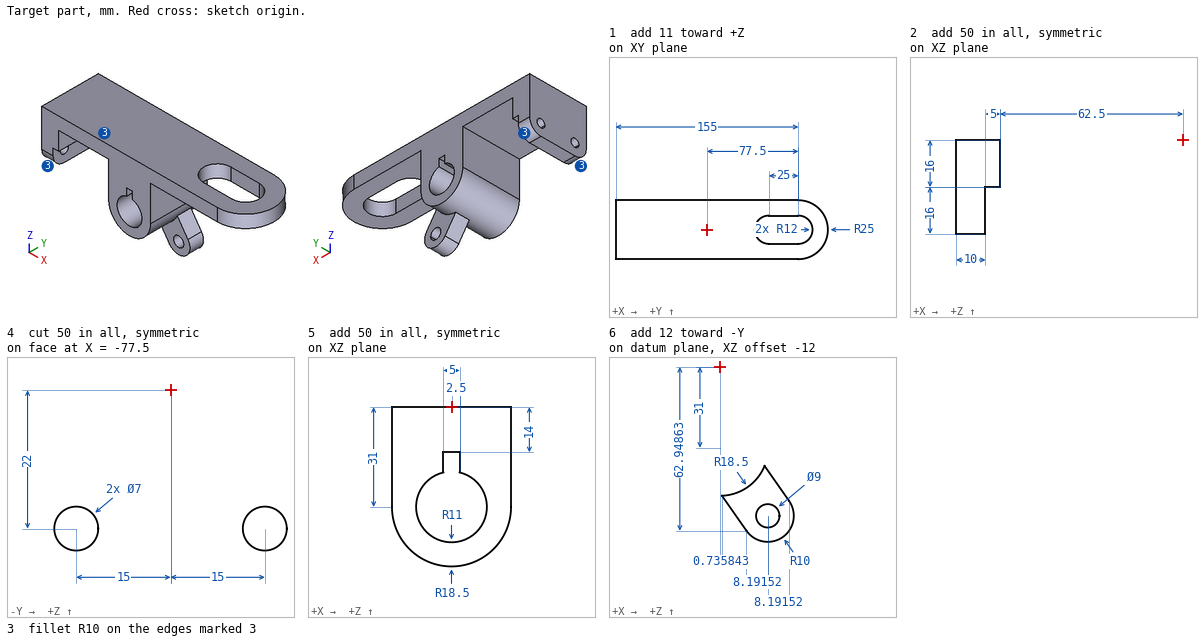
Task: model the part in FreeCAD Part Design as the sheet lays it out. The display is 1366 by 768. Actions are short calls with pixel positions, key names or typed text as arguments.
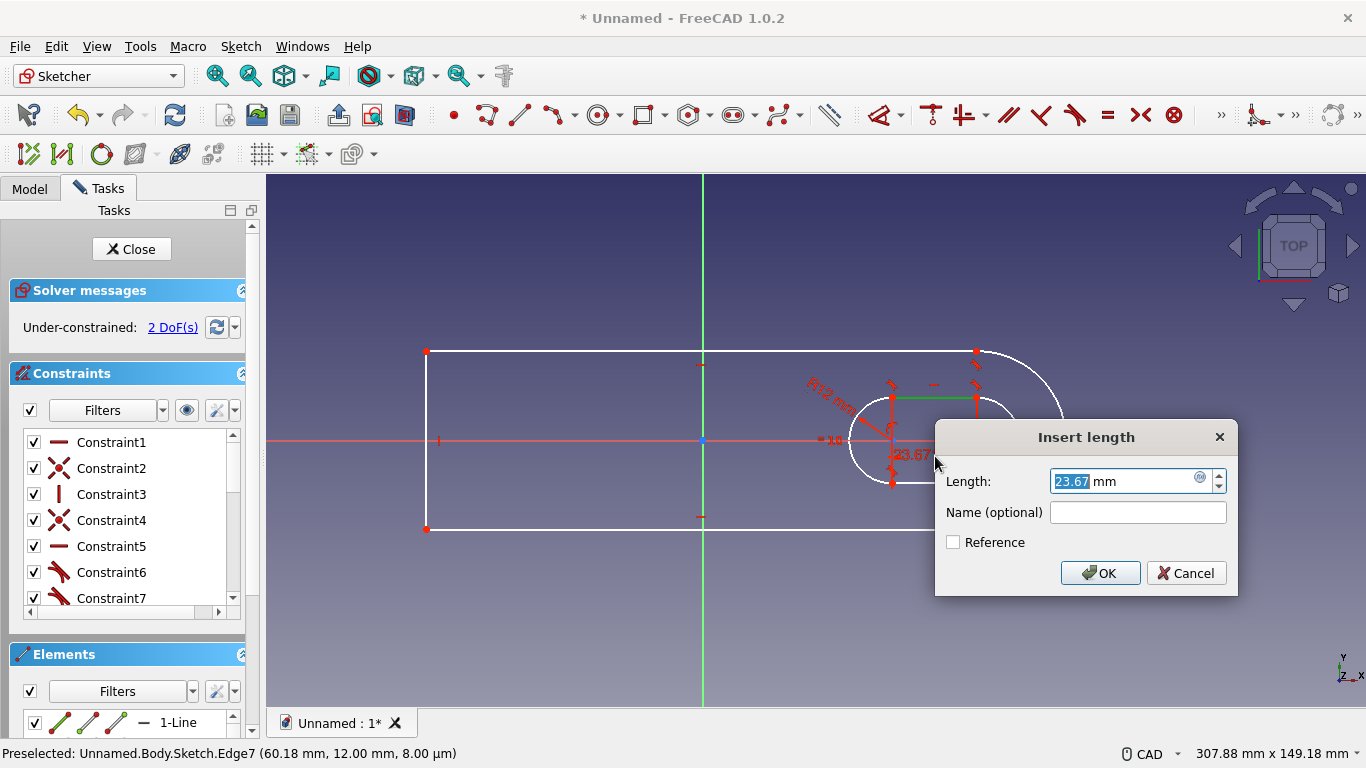
text(25)
key(Return)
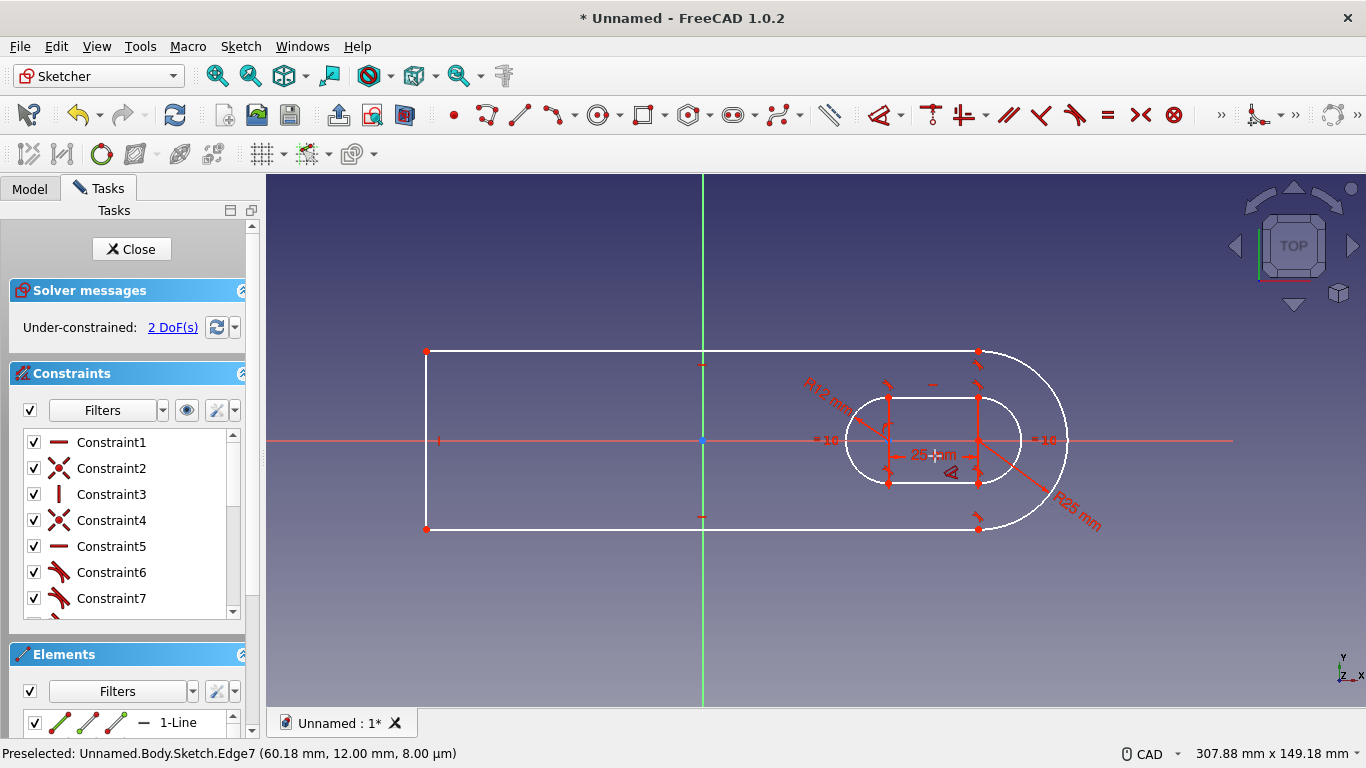
click(813, 351)
click(575, 317)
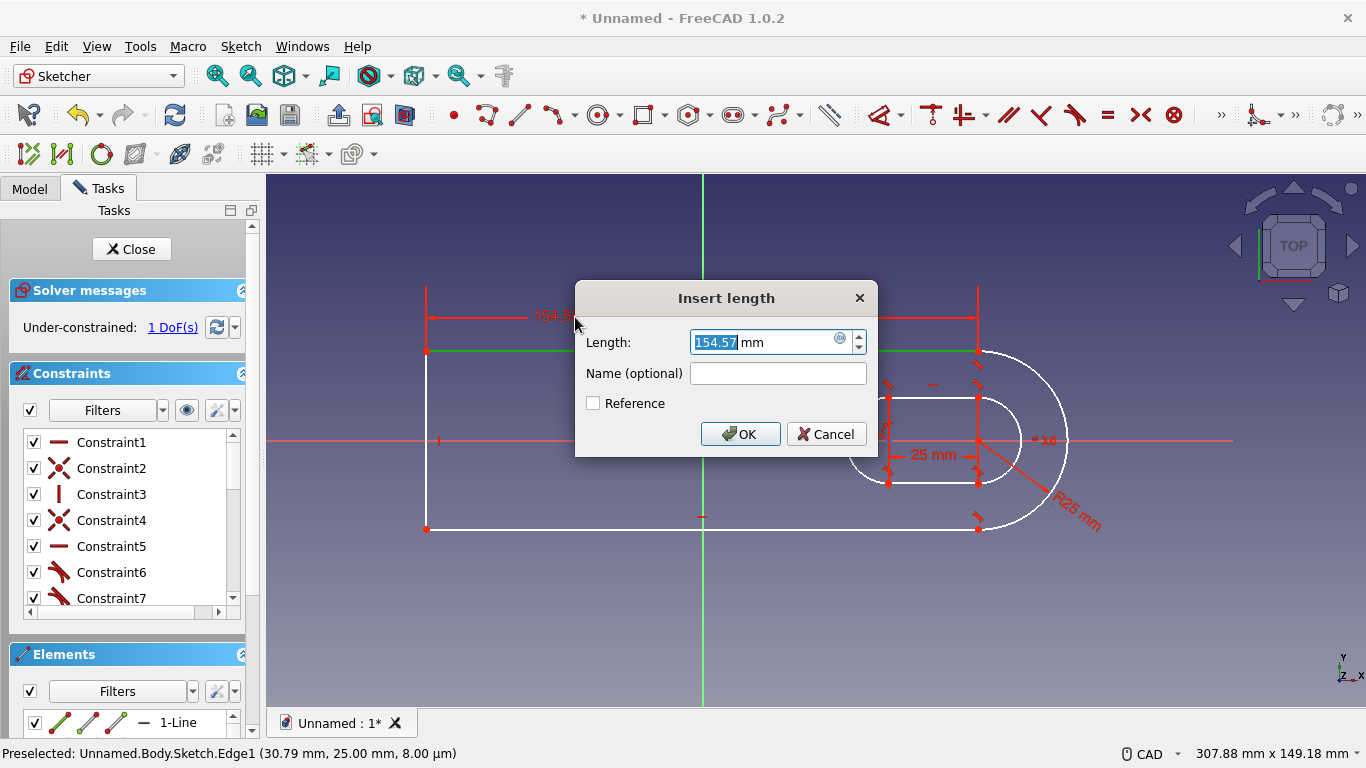
text(155)
key(Return)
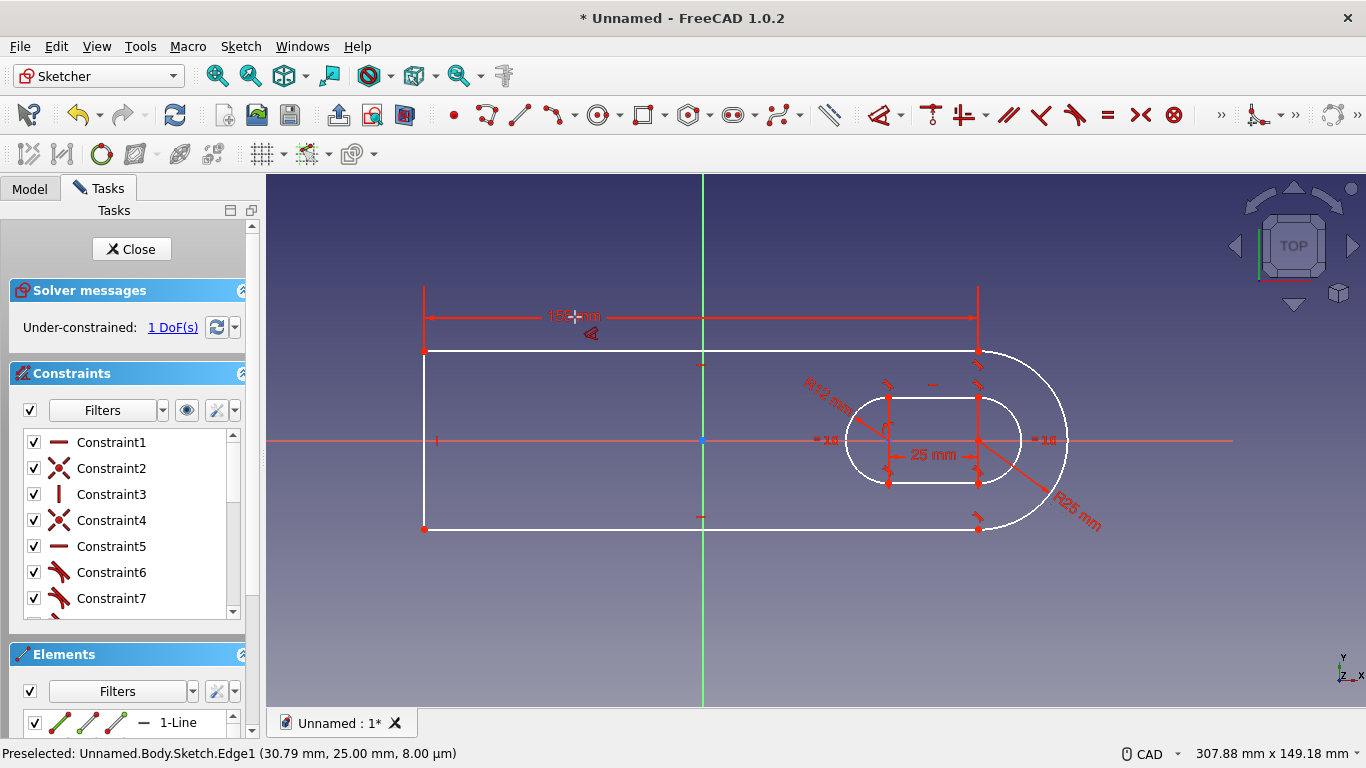
click(978, 351)
click(841, 317)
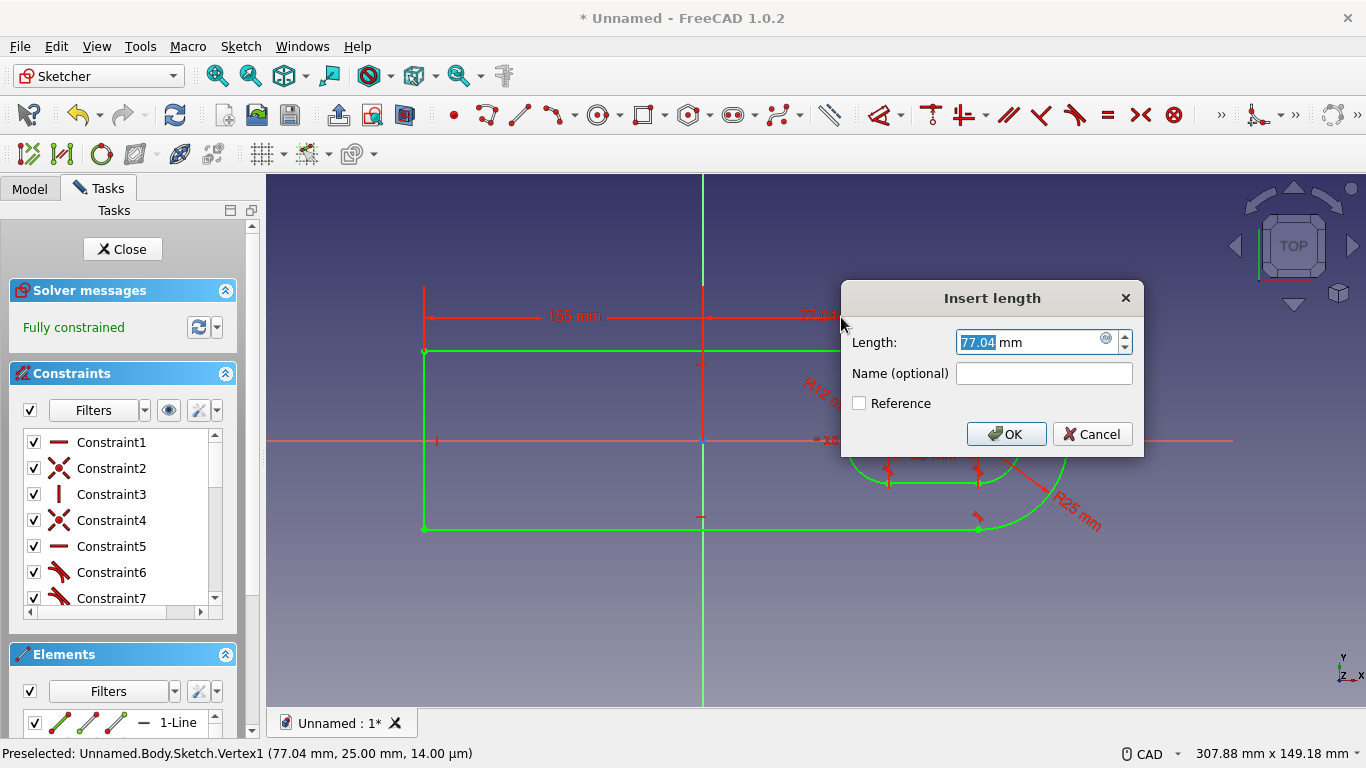
text(77.5)
key(Return)
key(Escape)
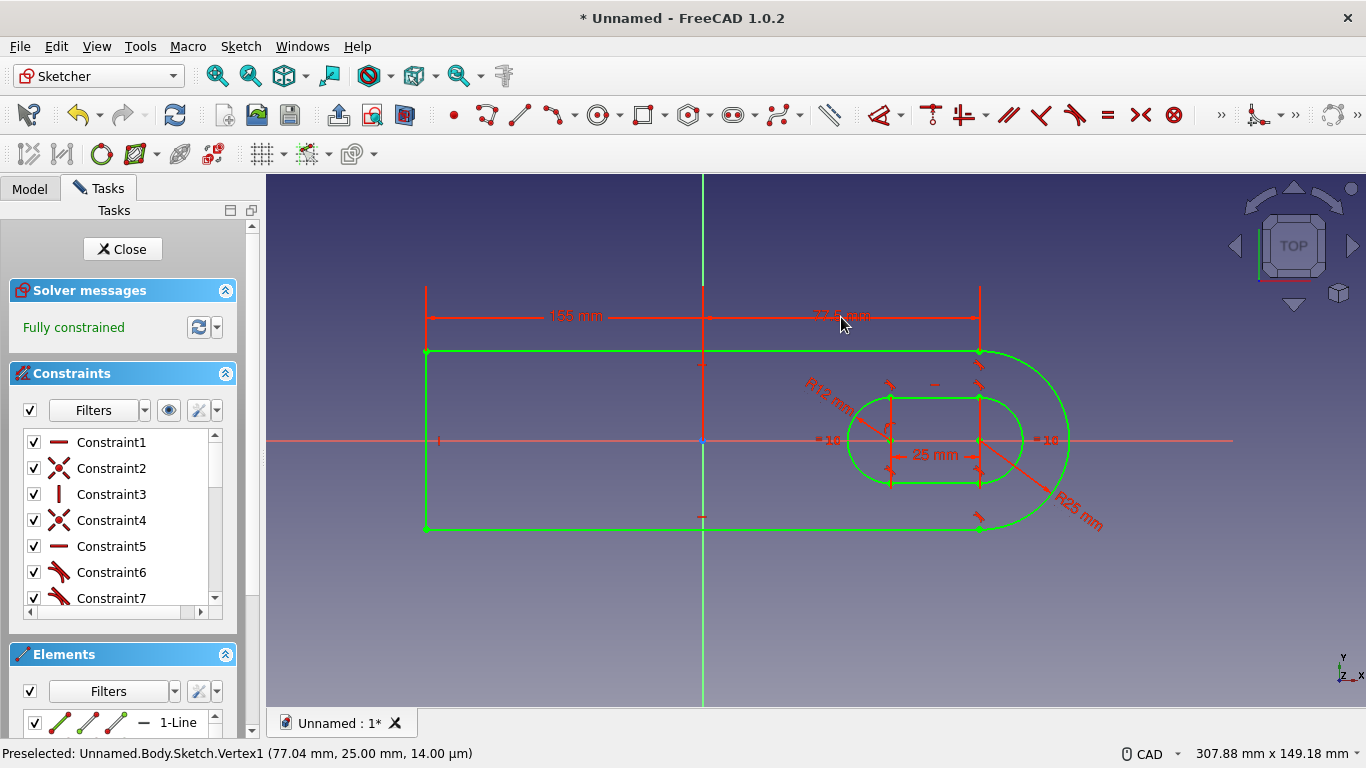
click(123, 249)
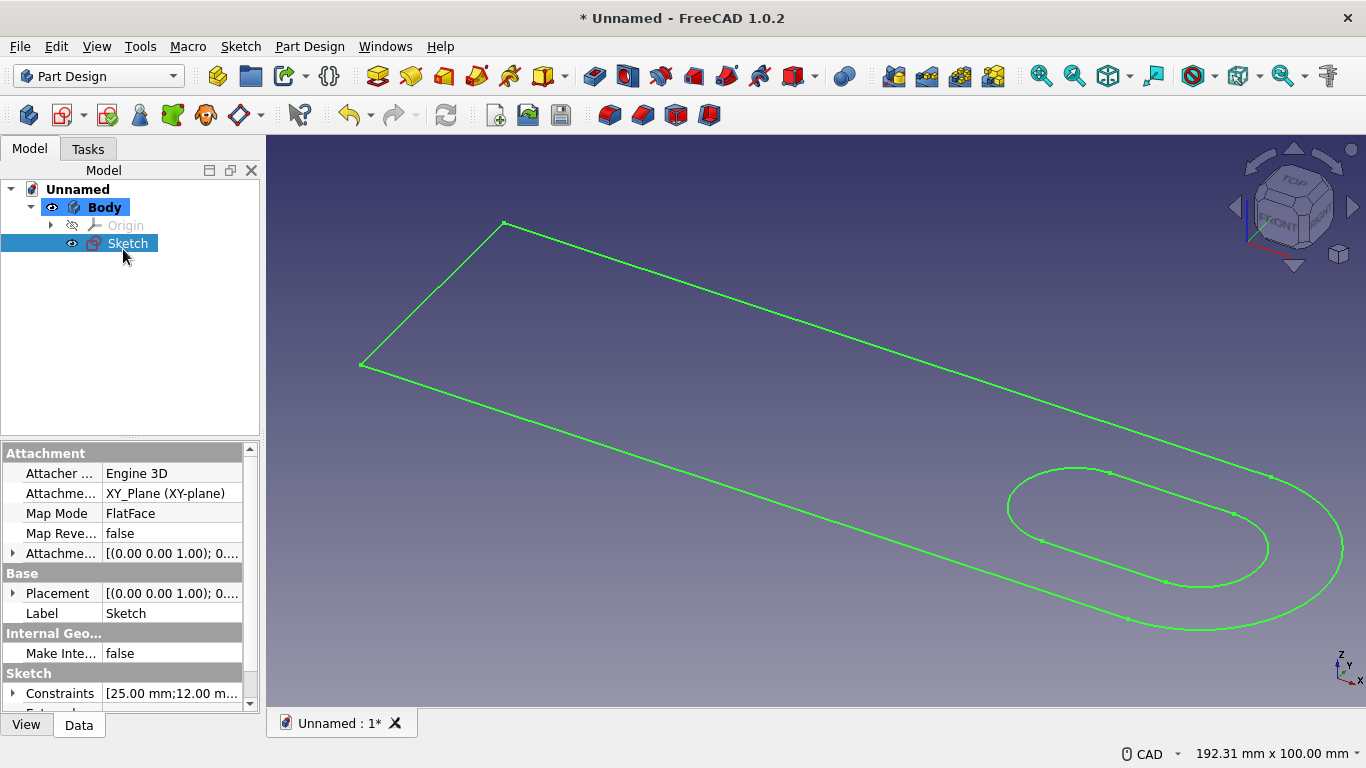
click(378, 76)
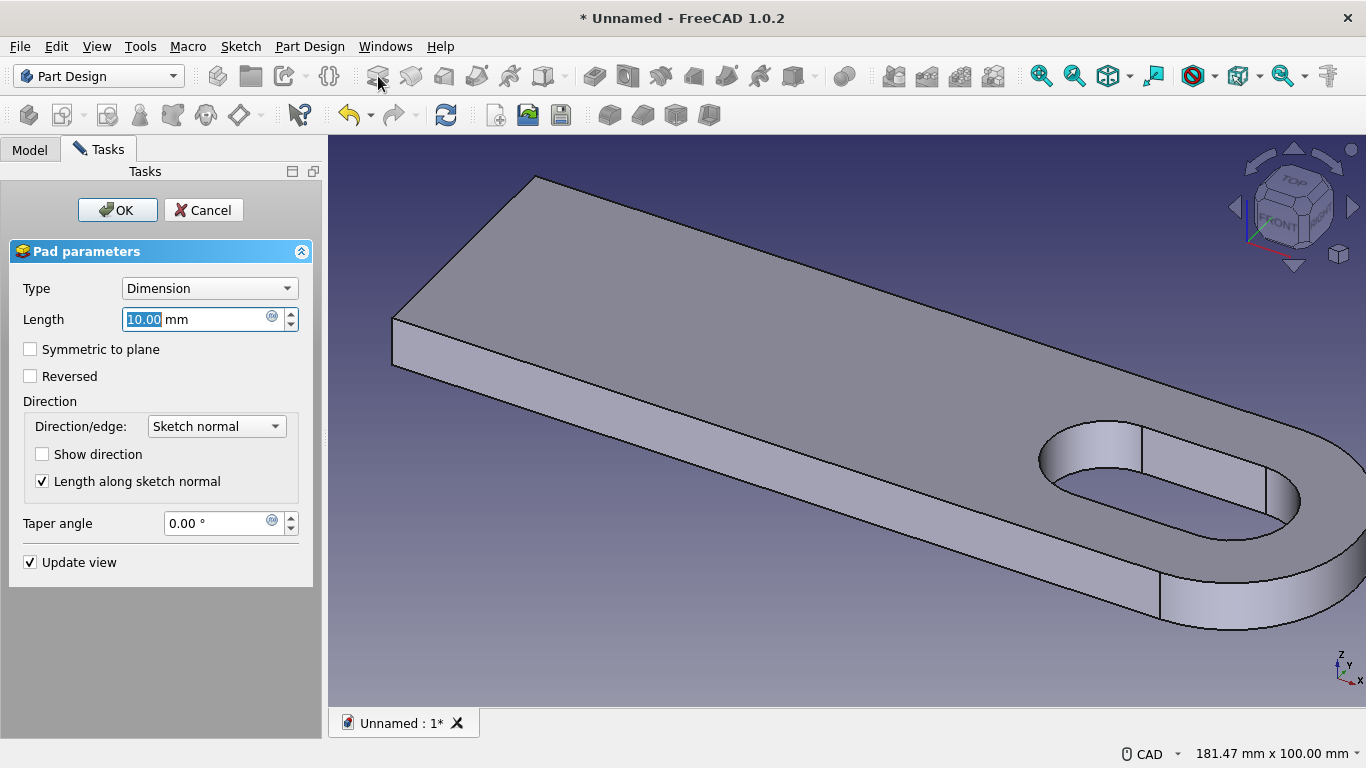
text(11)
key(Tab)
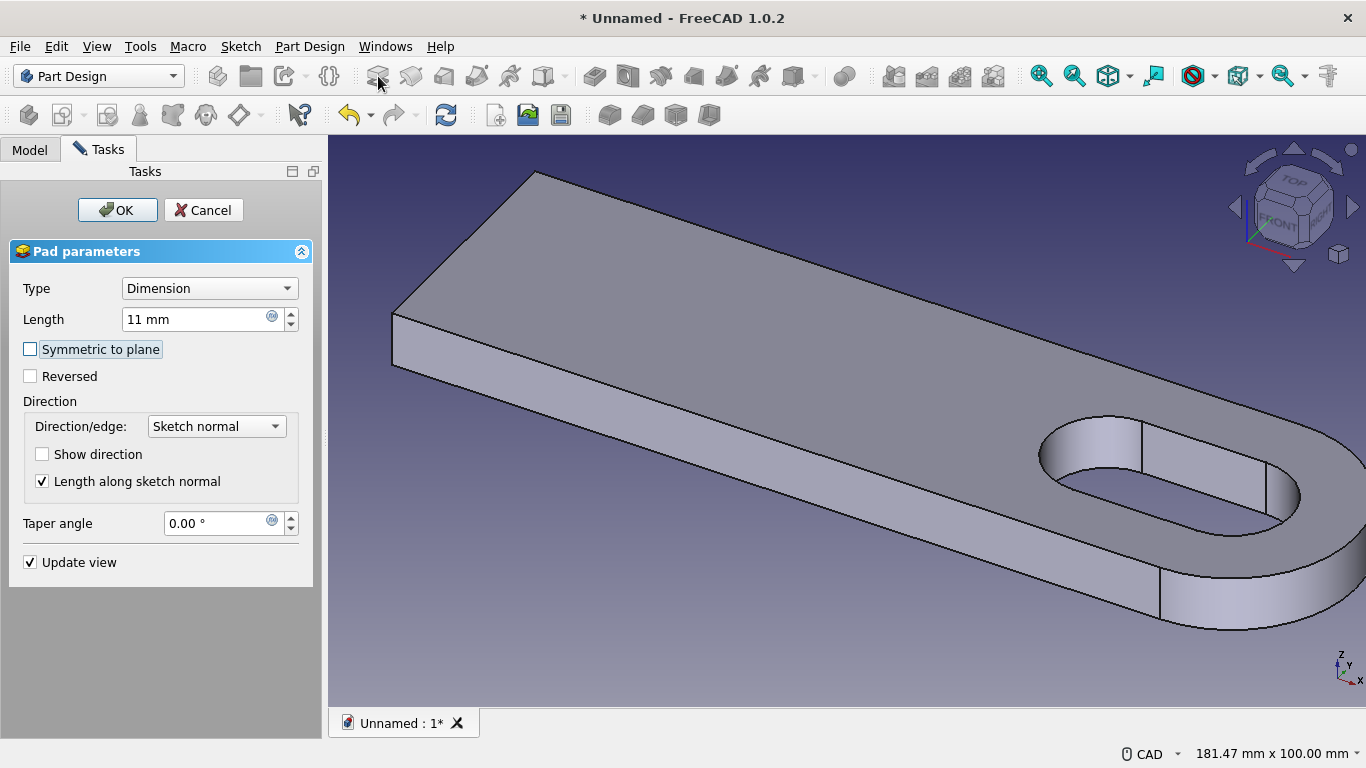
click(118, 210)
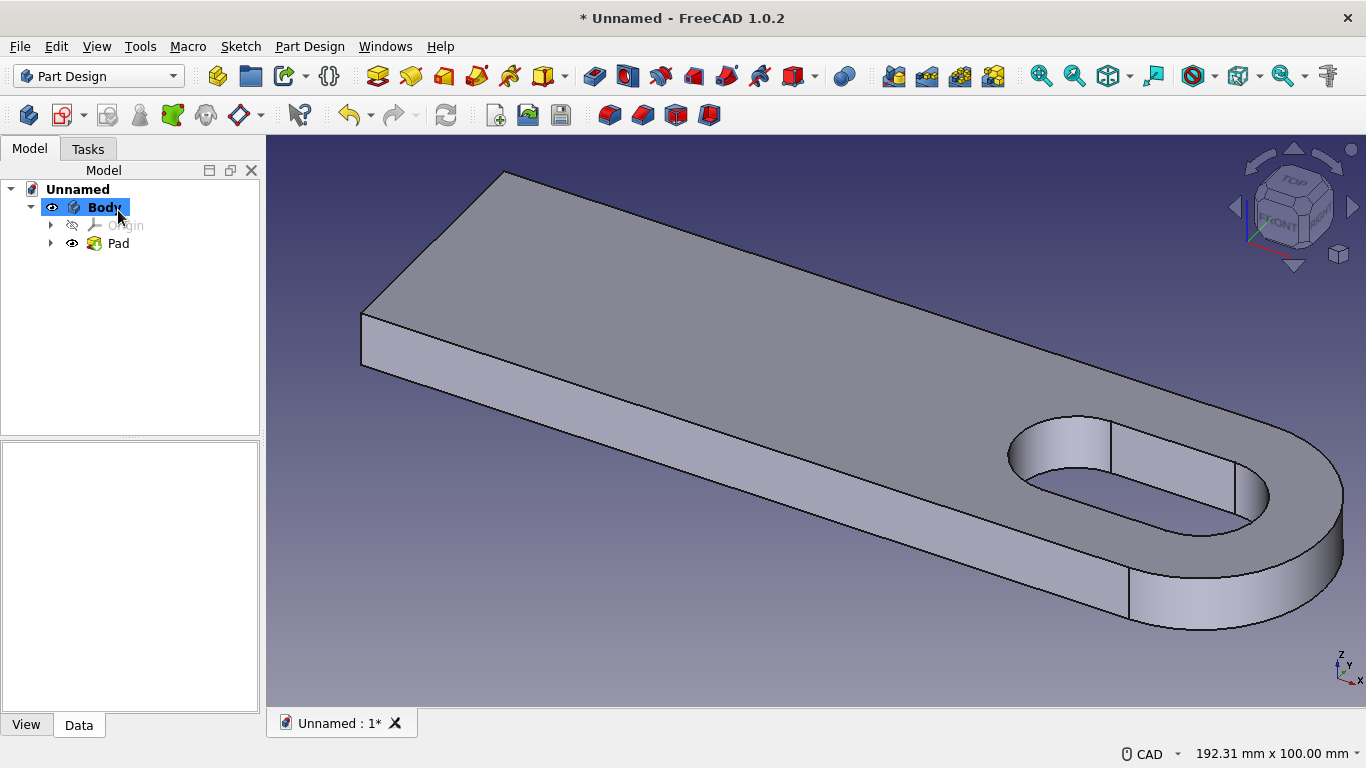
click(1042, 76)